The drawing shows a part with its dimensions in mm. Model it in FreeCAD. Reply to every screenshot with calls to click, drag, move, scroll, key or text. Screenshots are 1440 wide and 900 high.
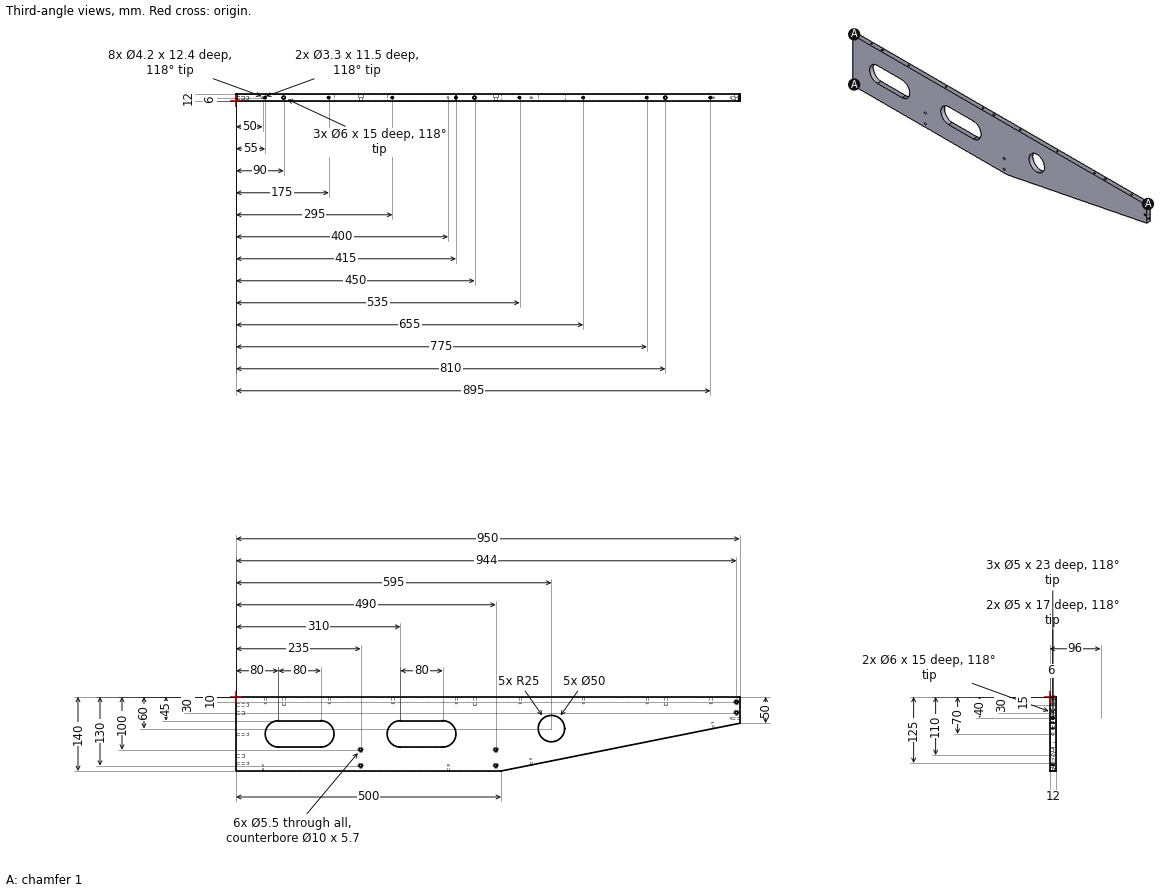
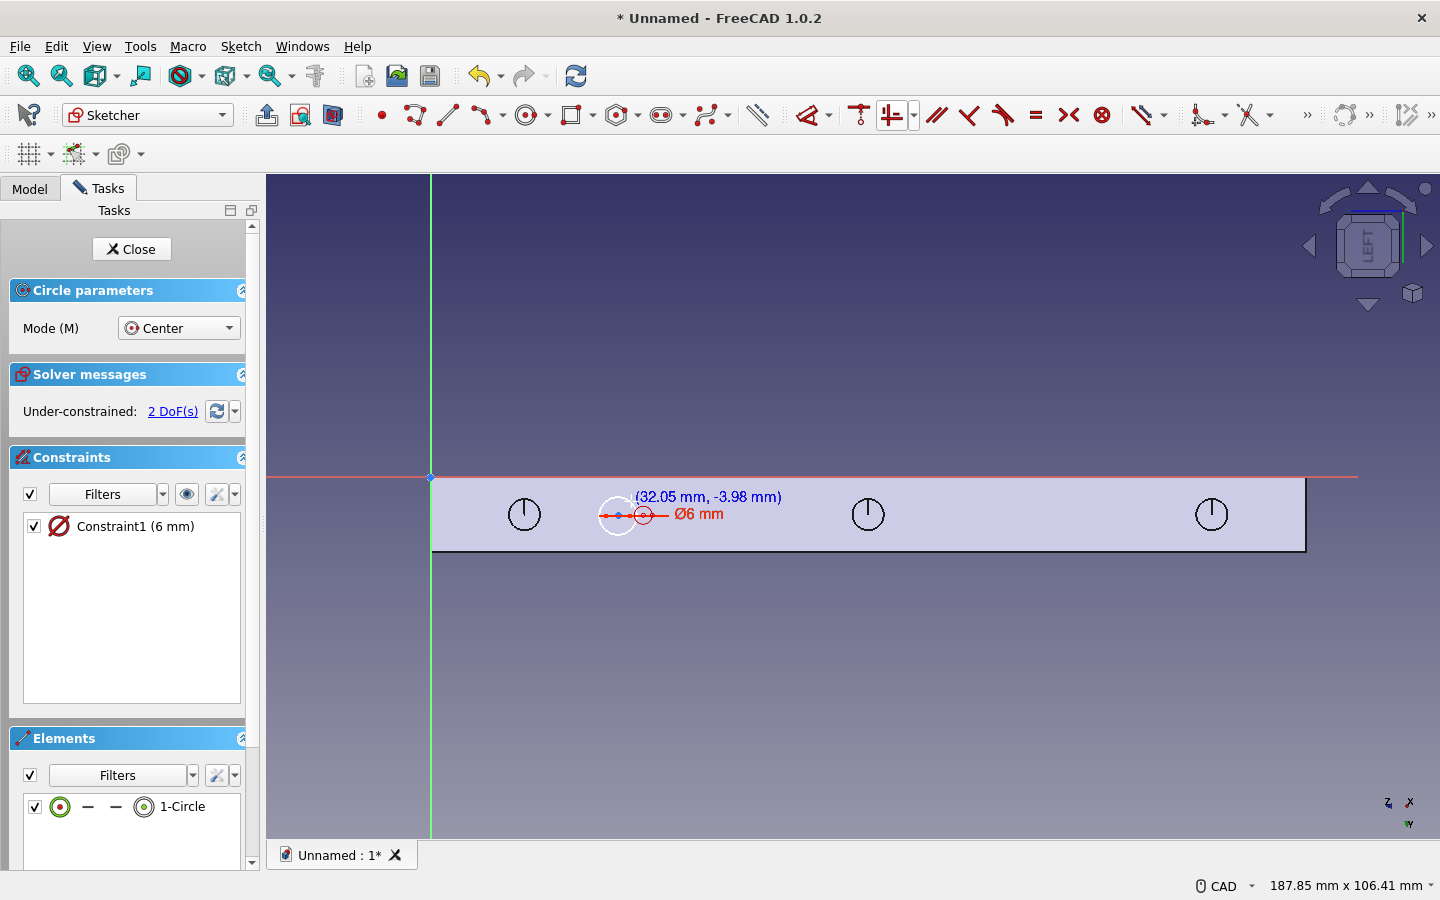
click(1118, 515)
move(1131, 501)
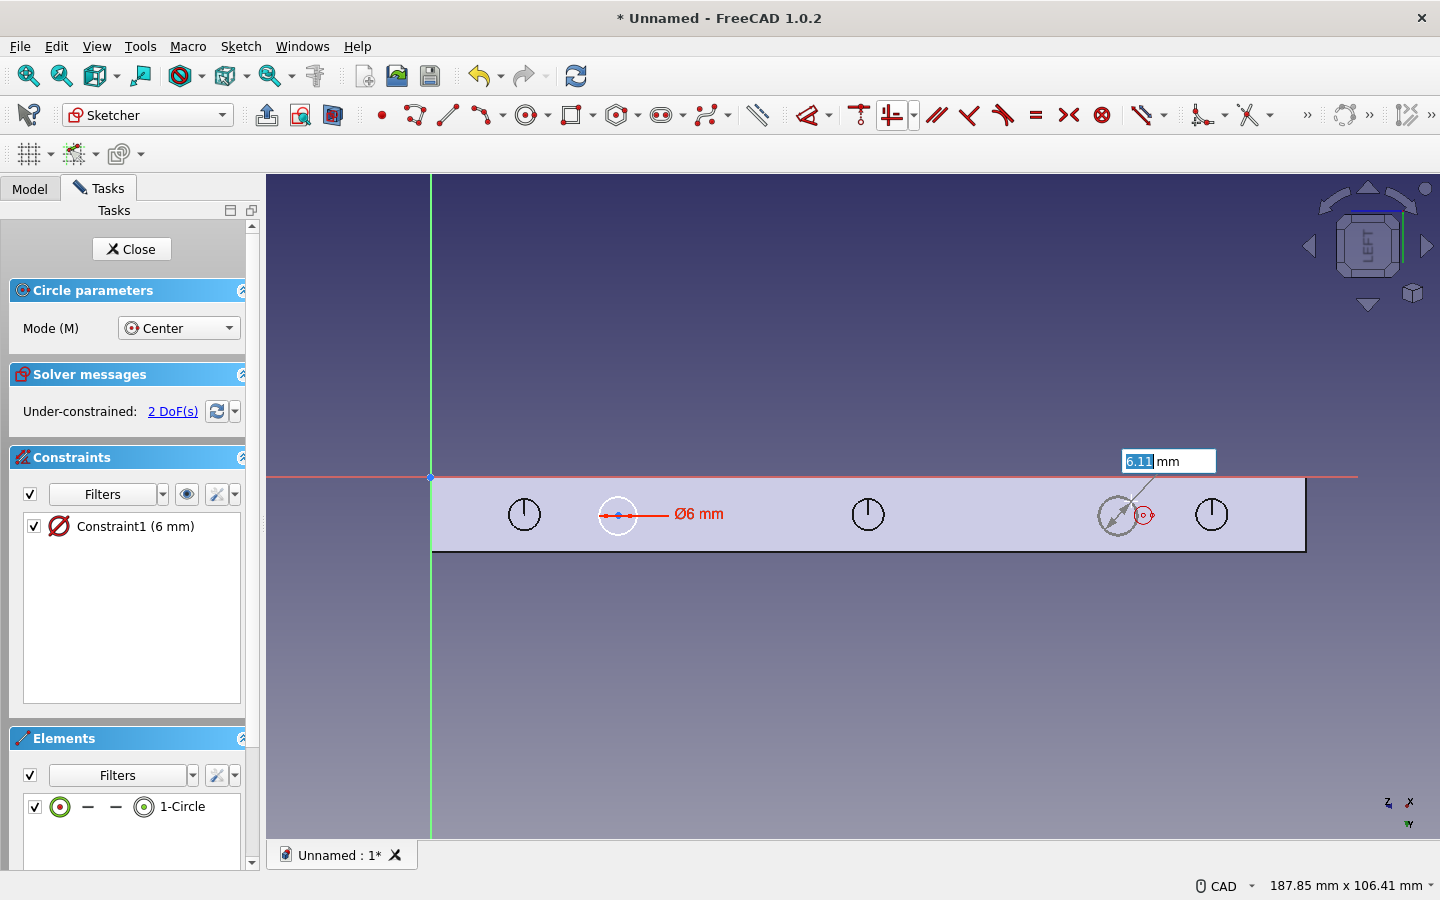
text(6)
key(Return)
key(Escape)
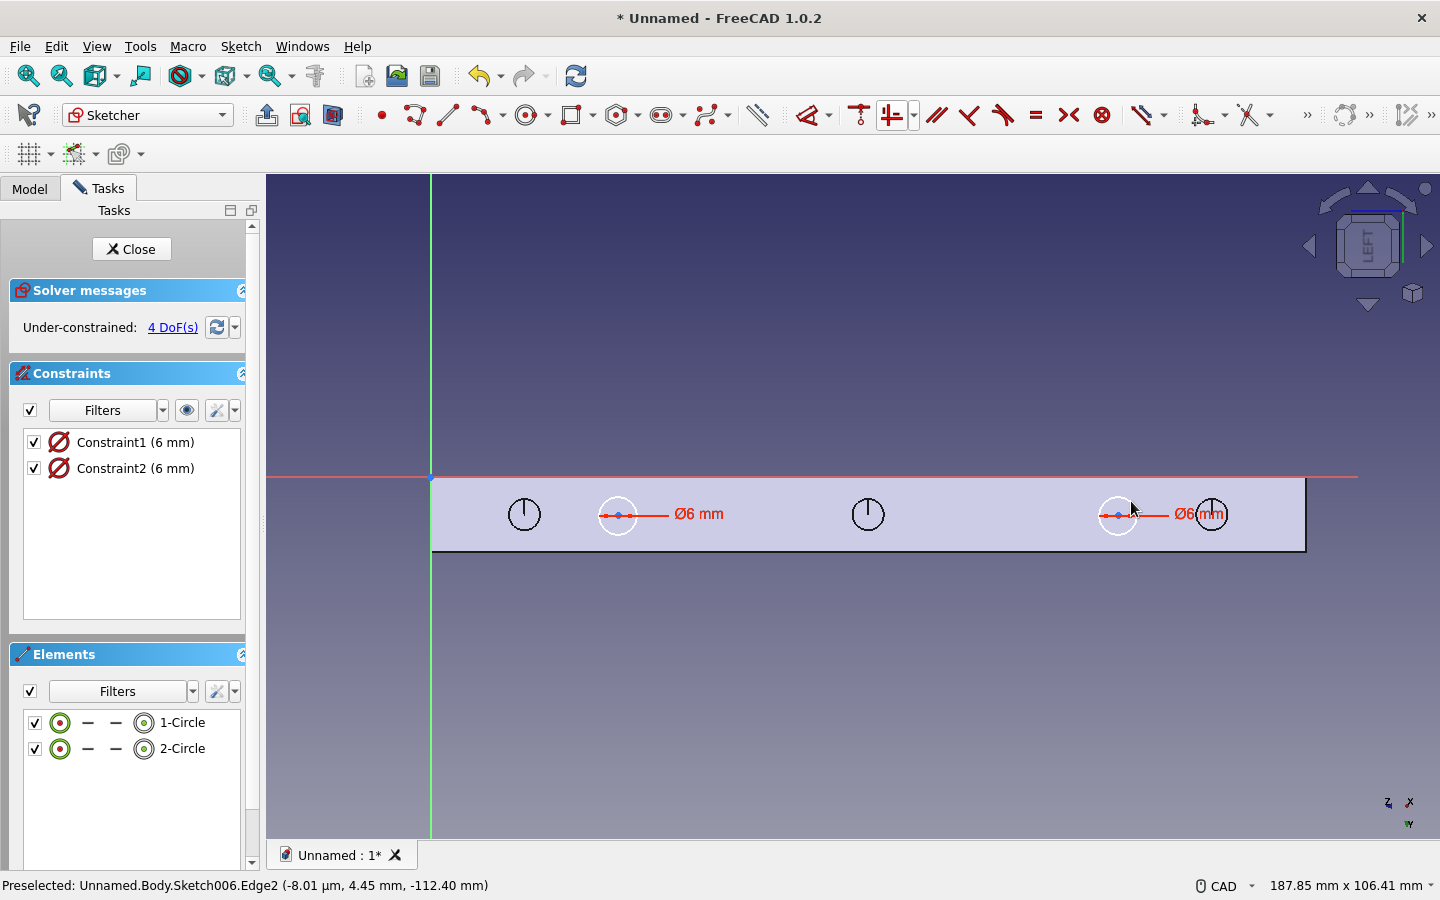
click(806, 116)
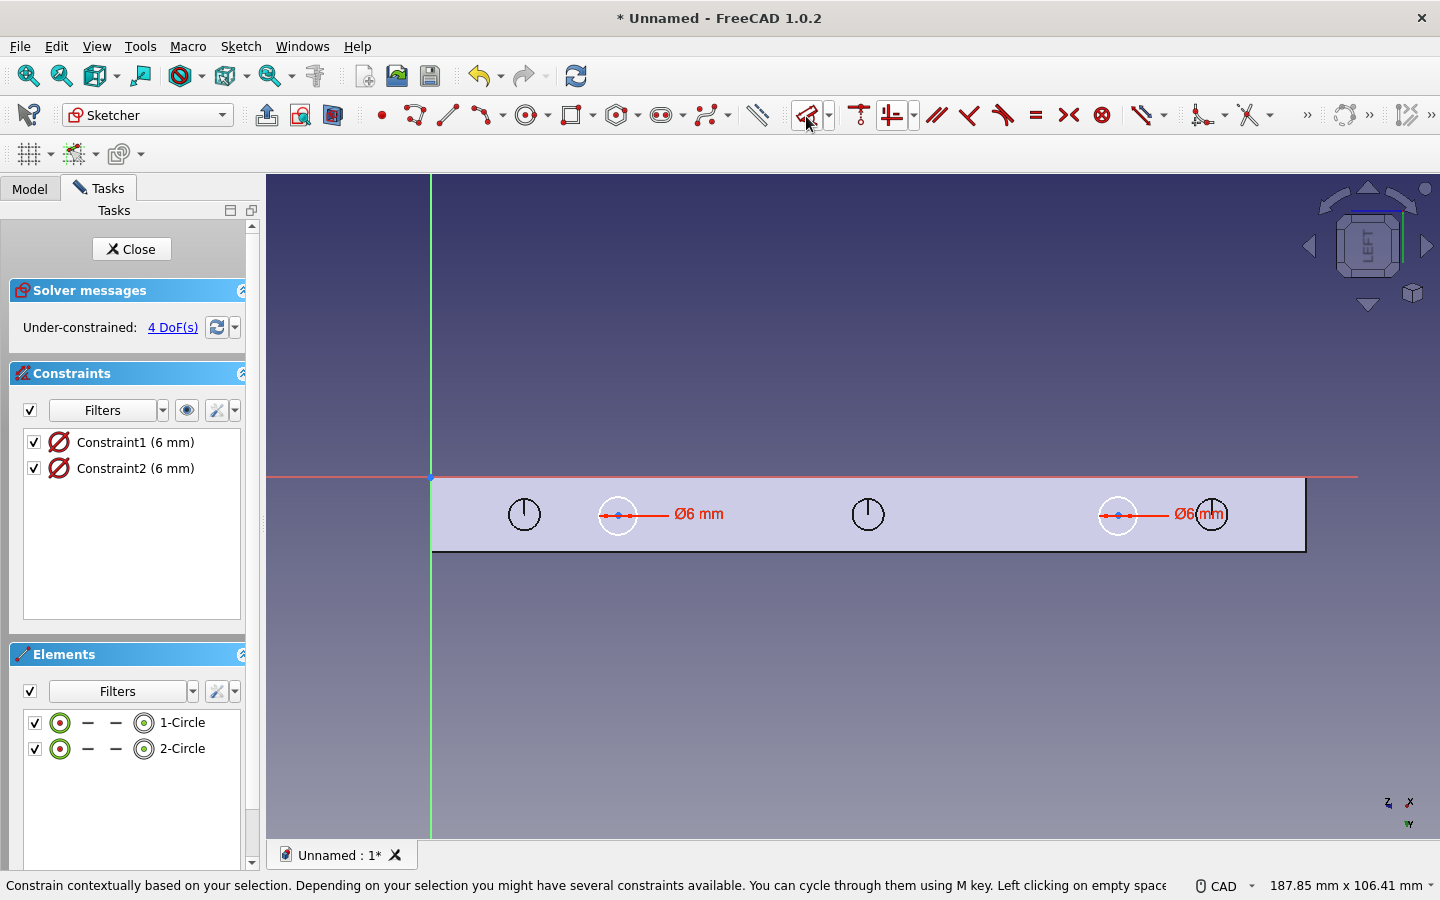
click(618, 516)
click(397, 497)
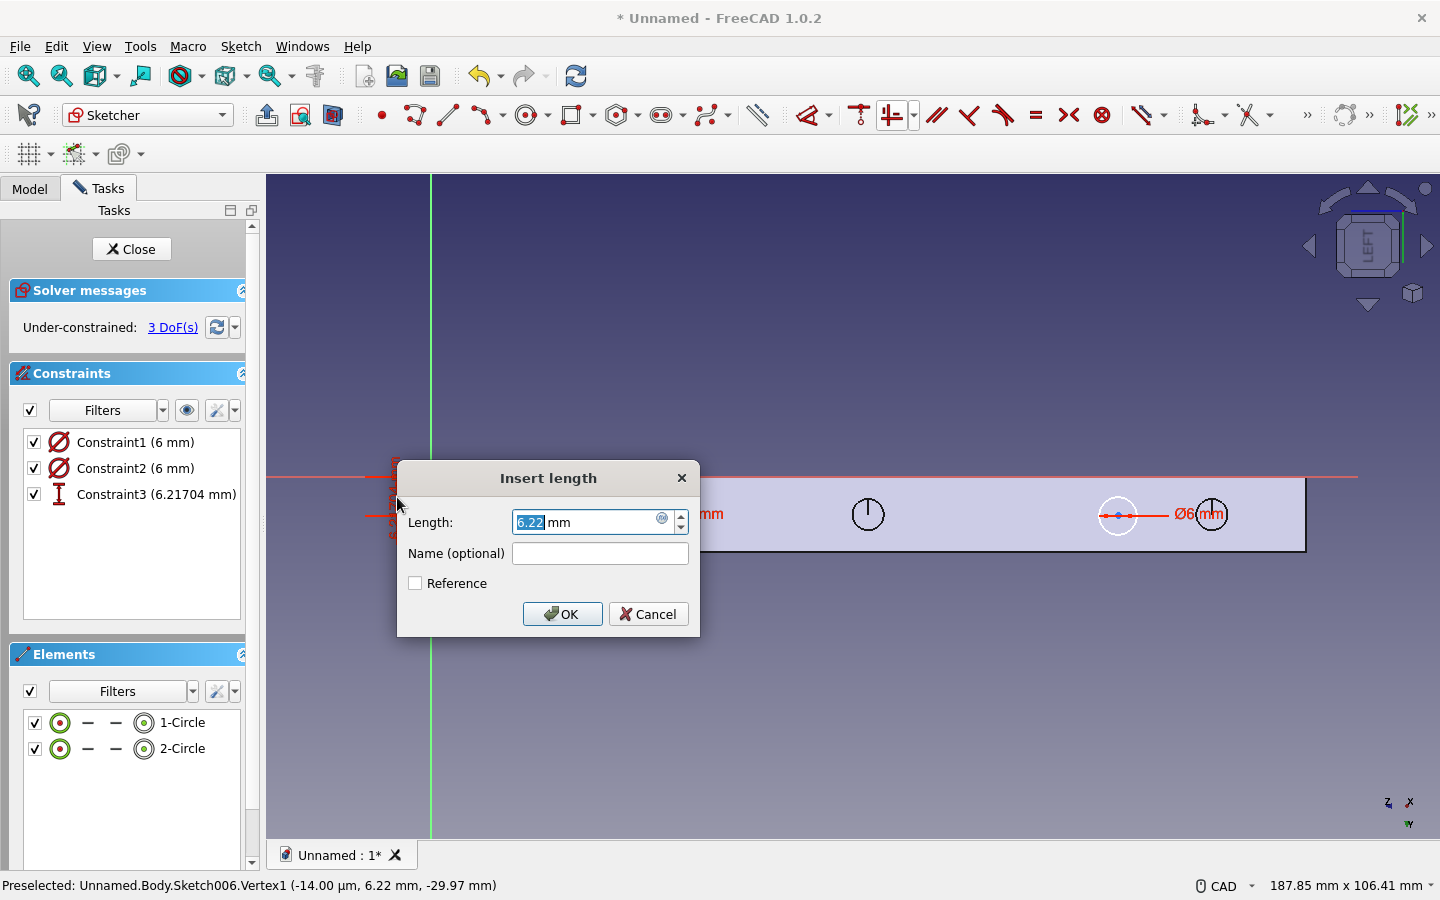
text(6)
key(Return)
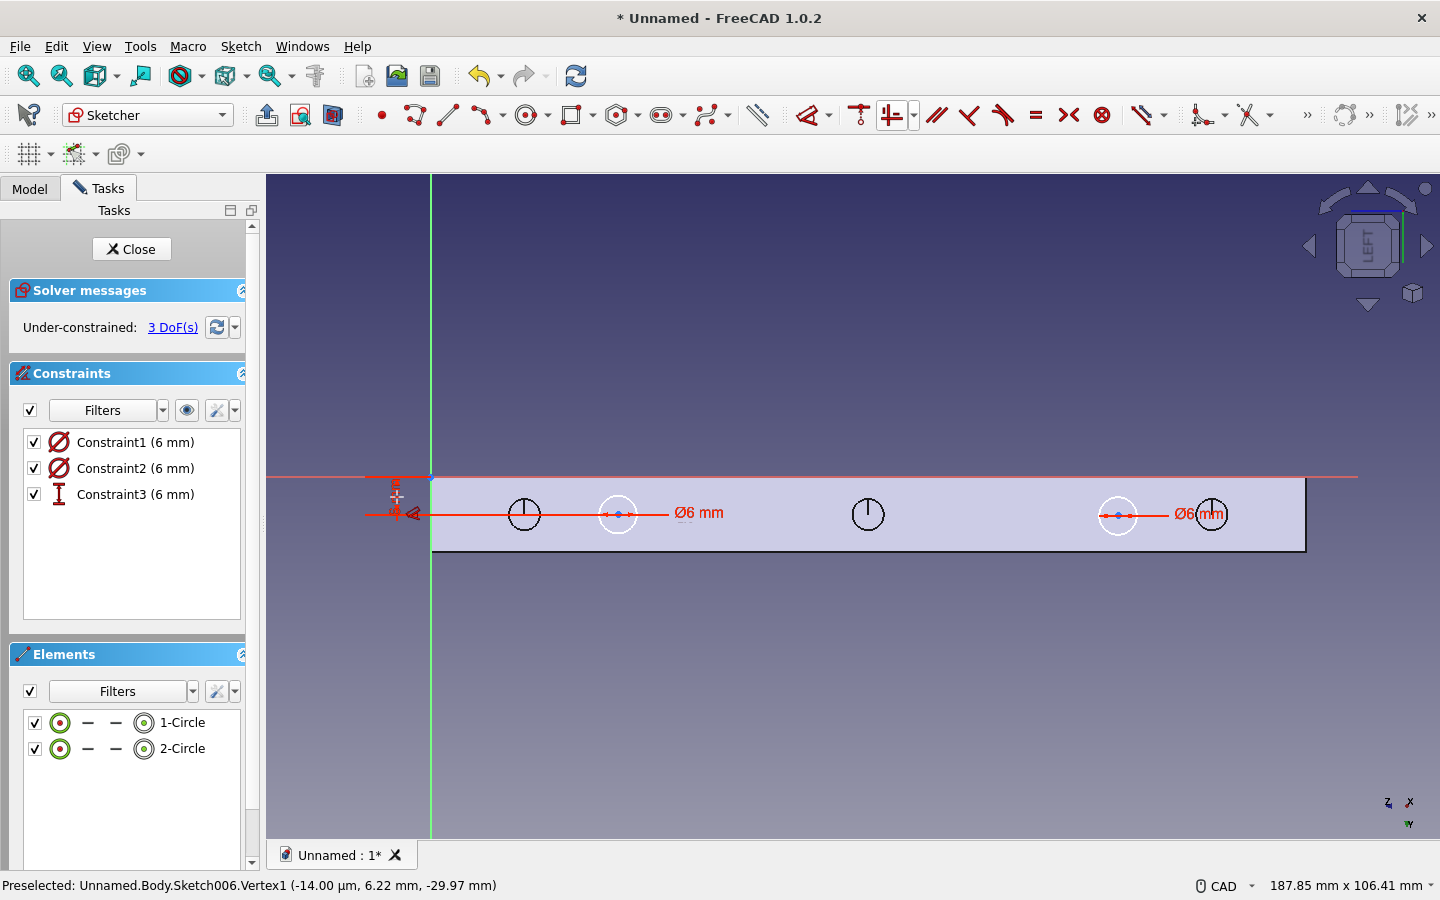
click(1118, 516)
click(1152, 497)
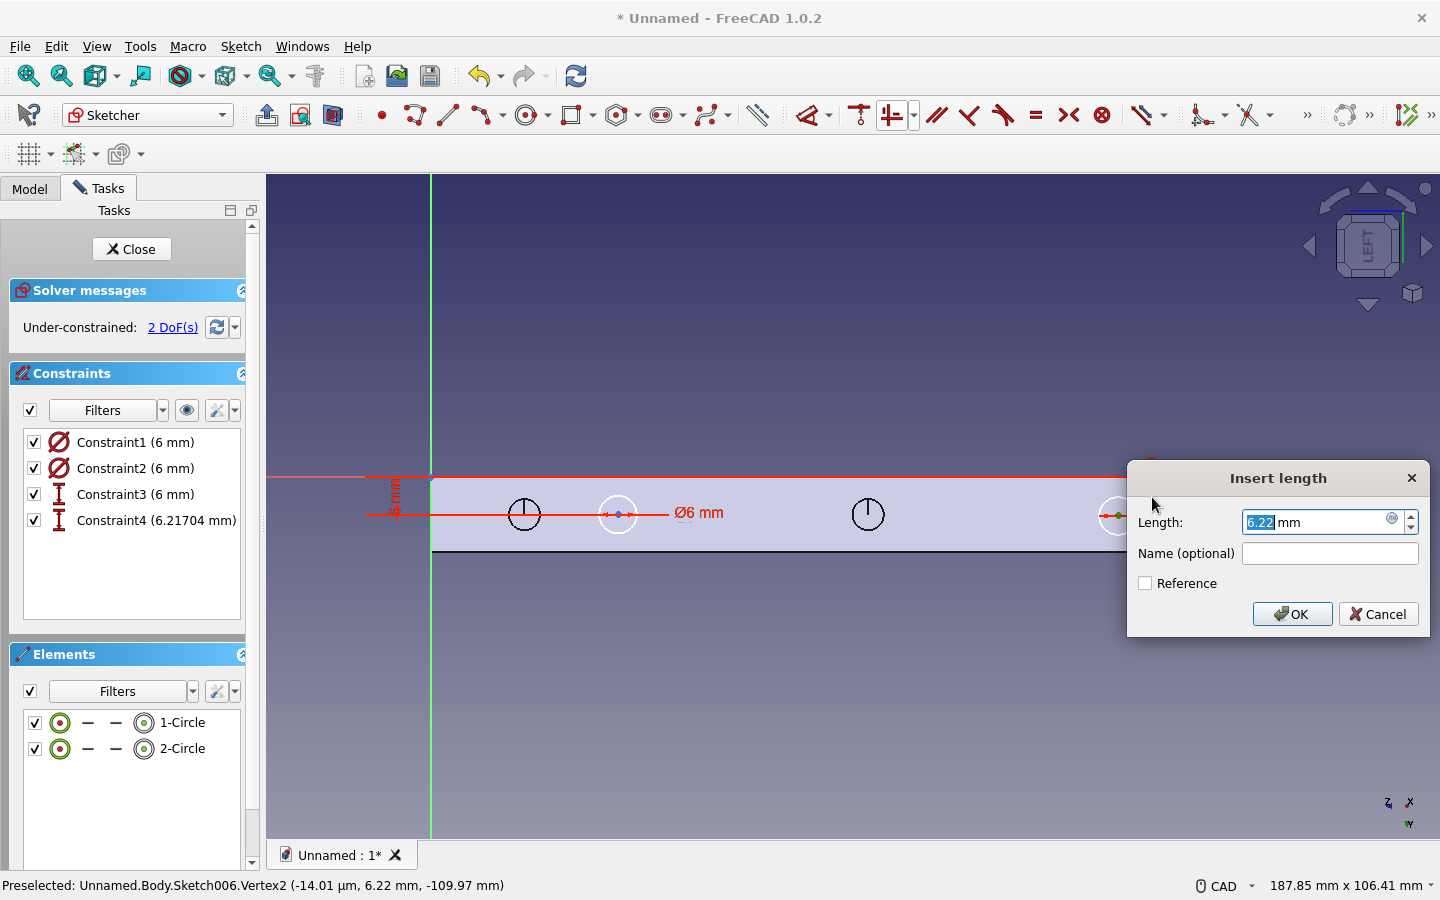
text(6)
key(Return)